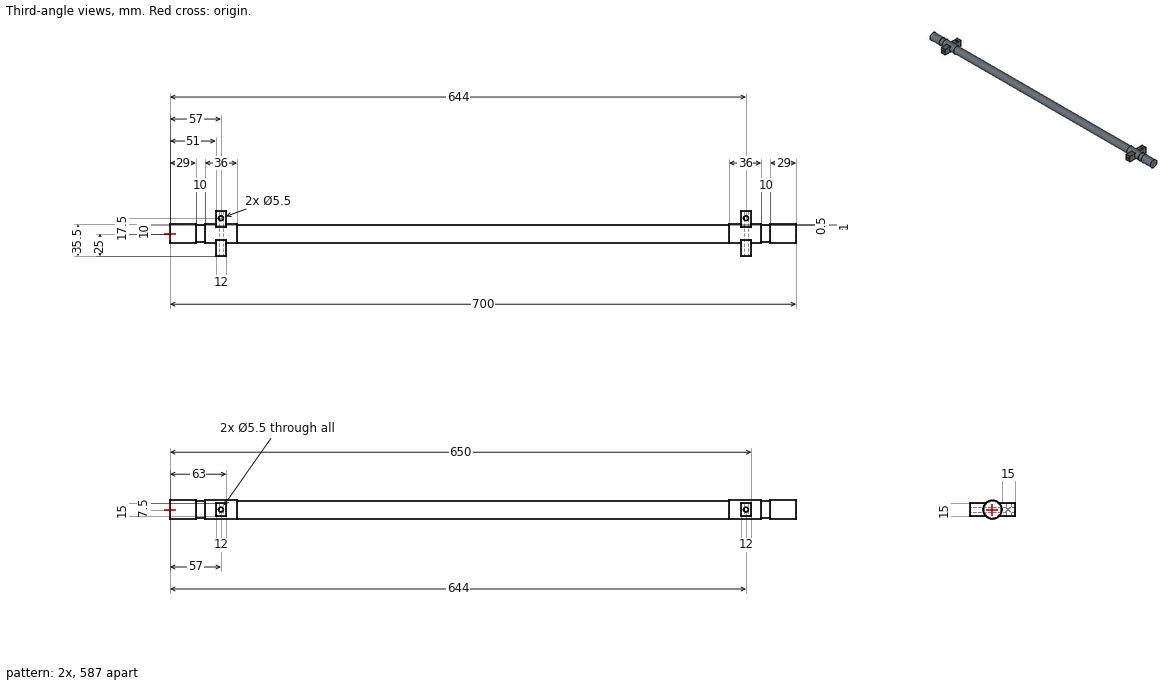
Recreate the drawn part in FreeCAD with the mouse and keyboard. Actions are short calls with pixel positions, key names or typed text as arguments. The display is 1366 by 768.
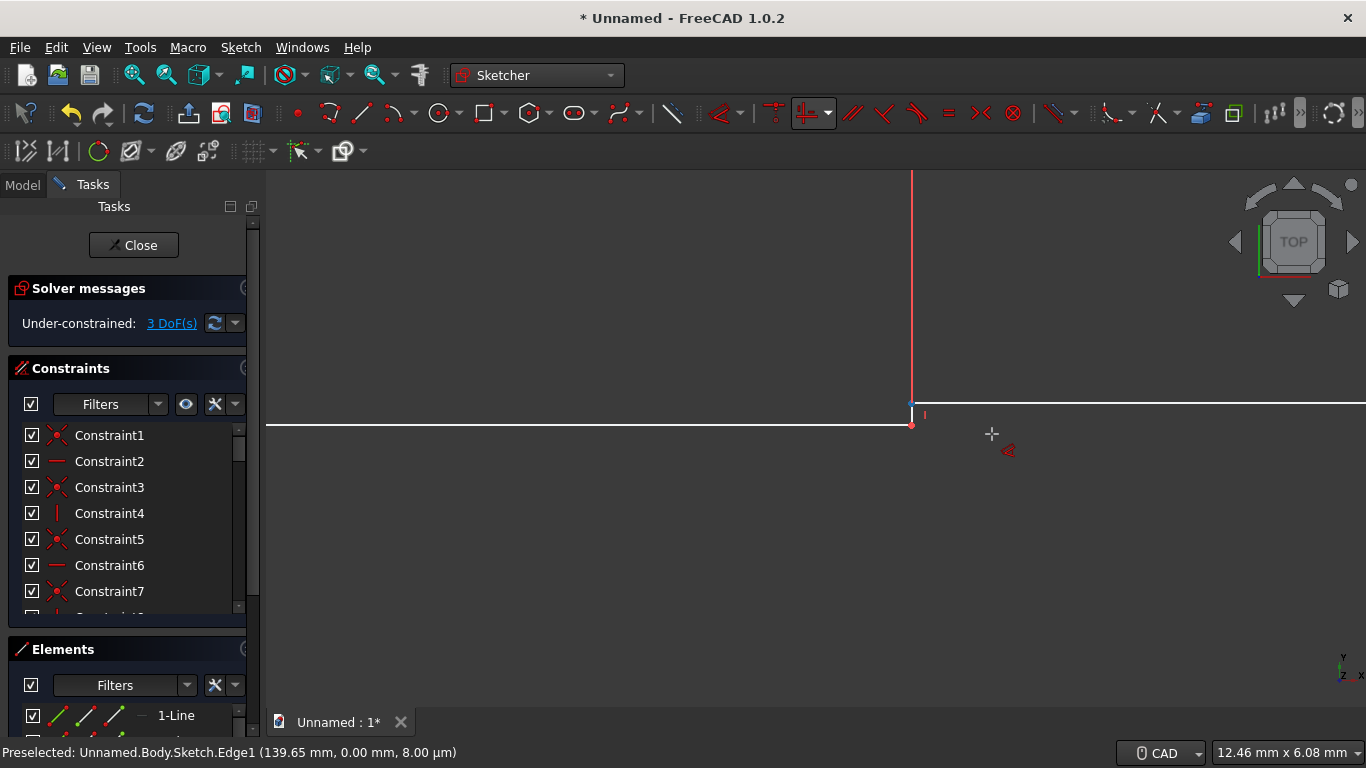
click(912, 414)
click(946, 419)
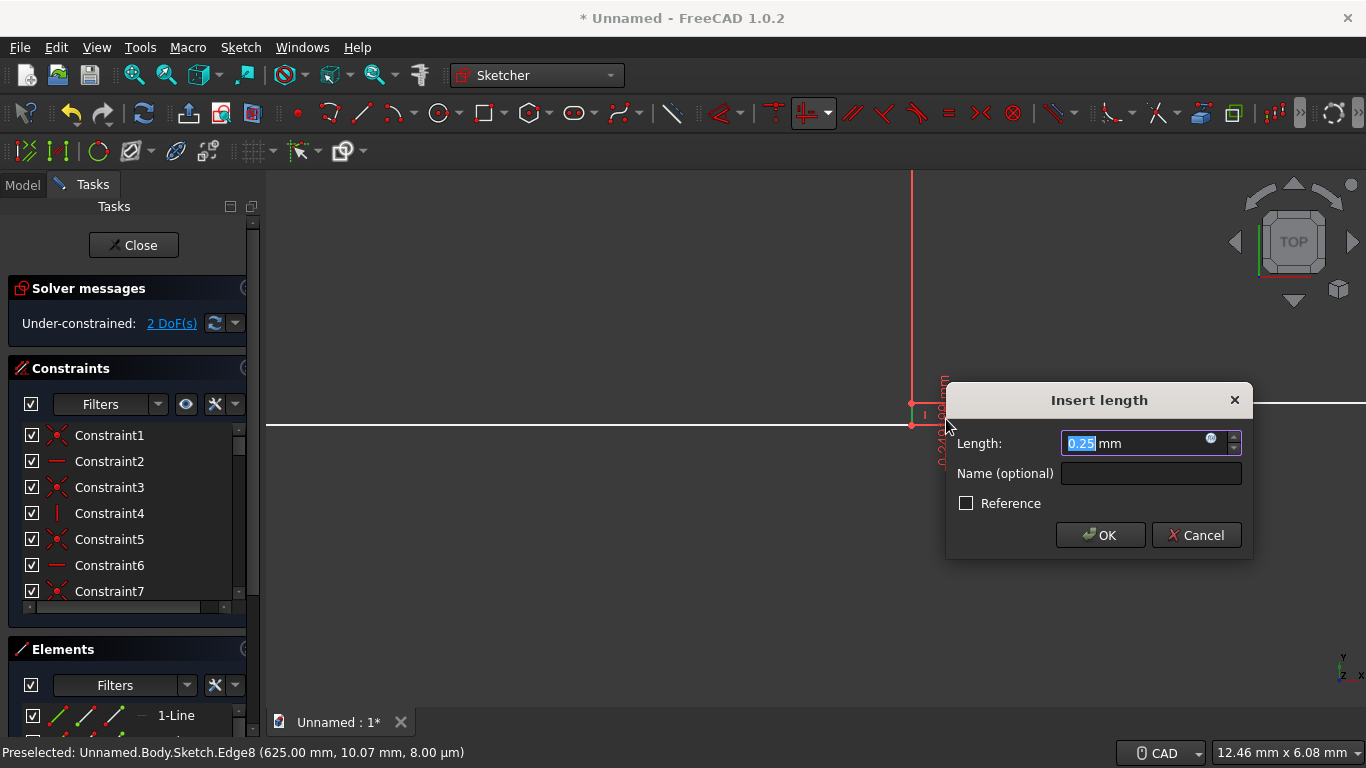
text(0.5)
key(Return)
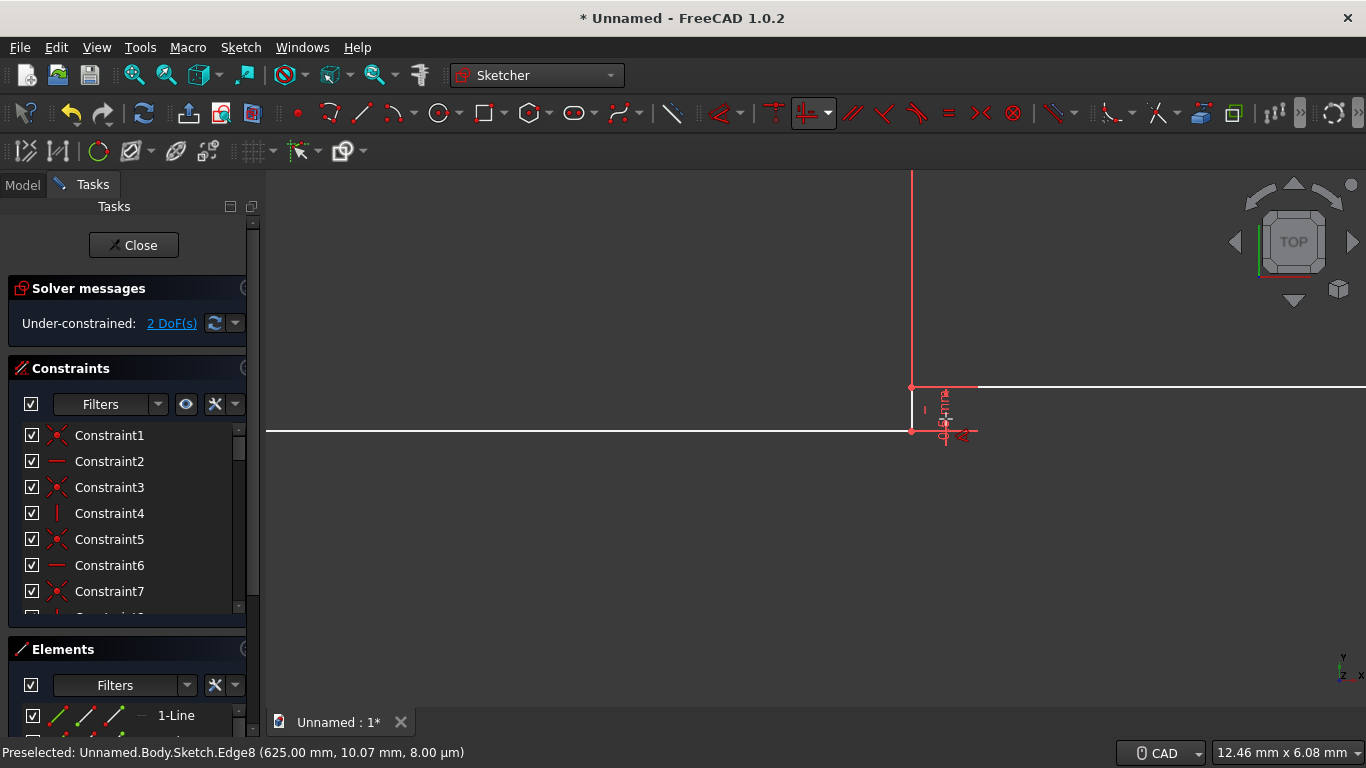
scroll(748, 438, down, 15)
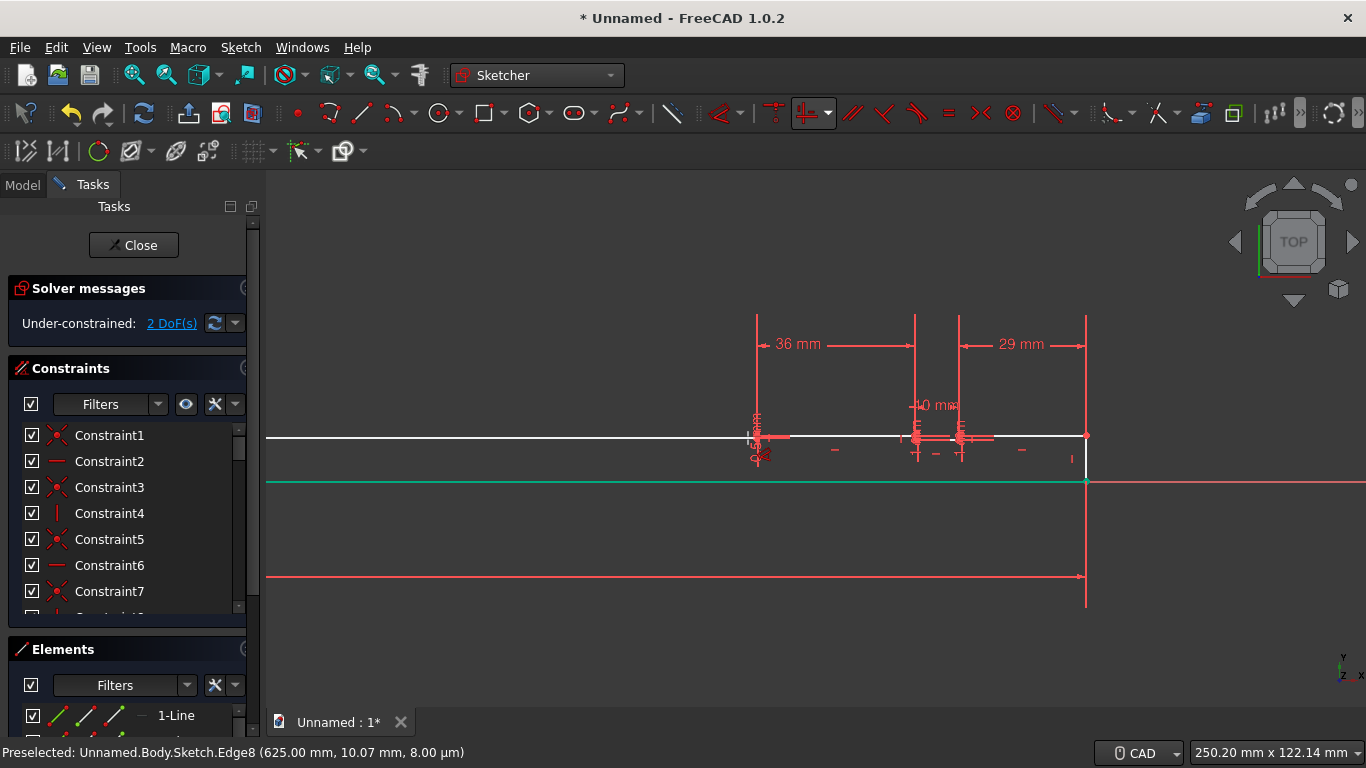
scroll(1051, 433, down, 8)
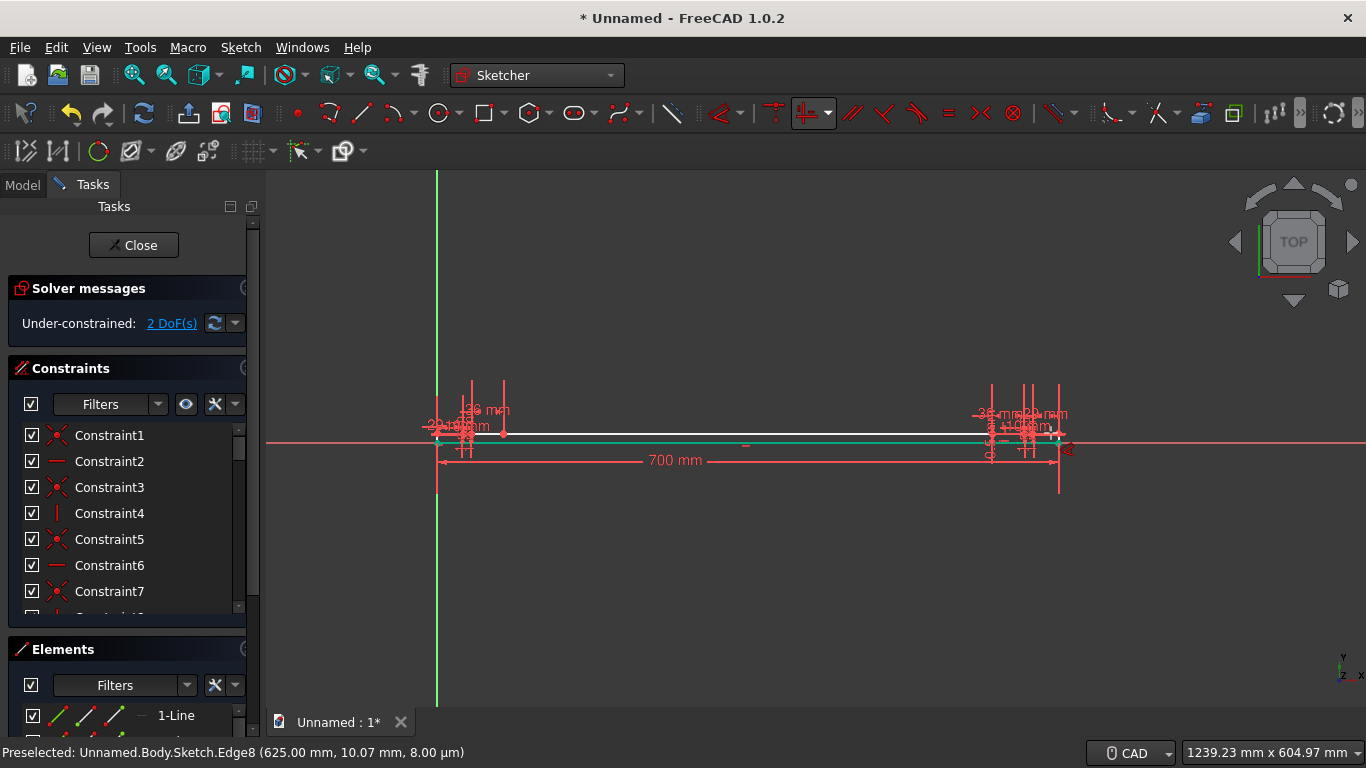
scroll(504, 434, up, 23)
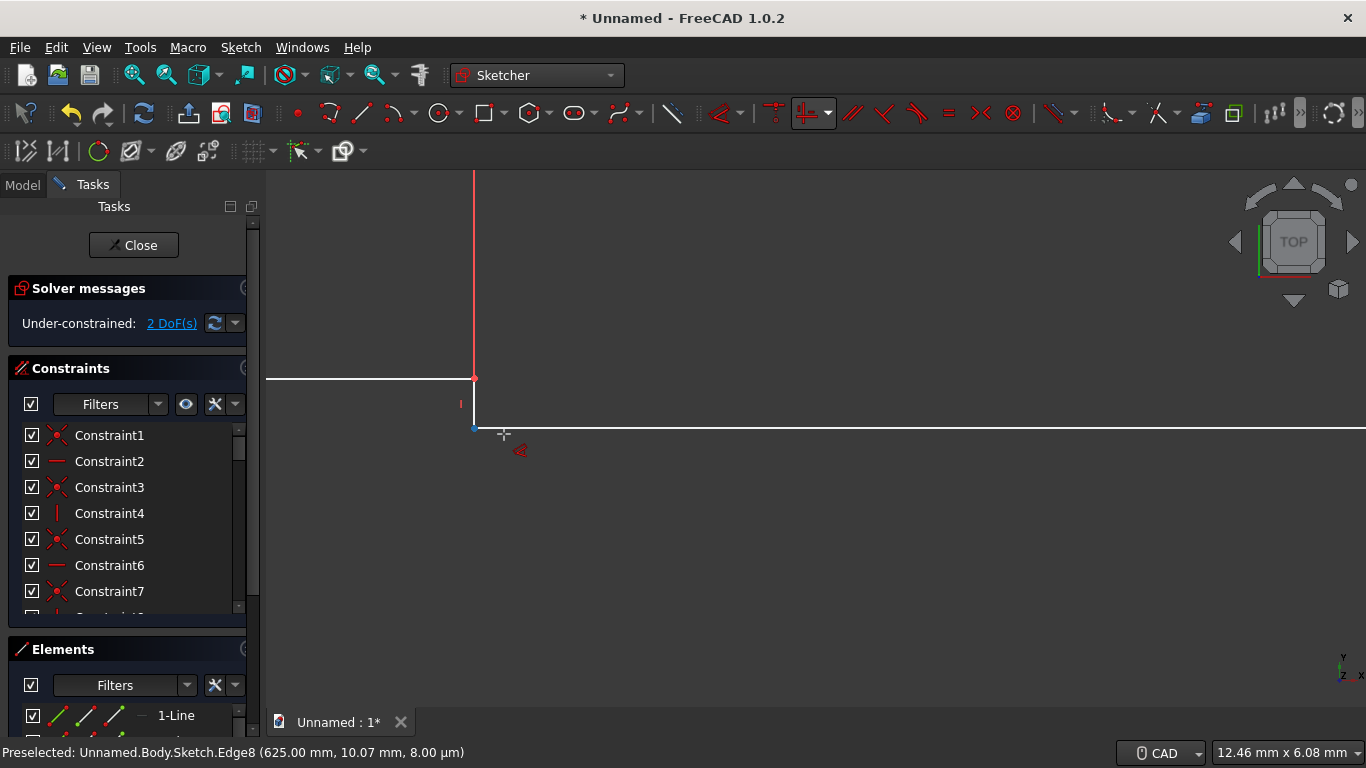
click(474, 413)
click(440, 403)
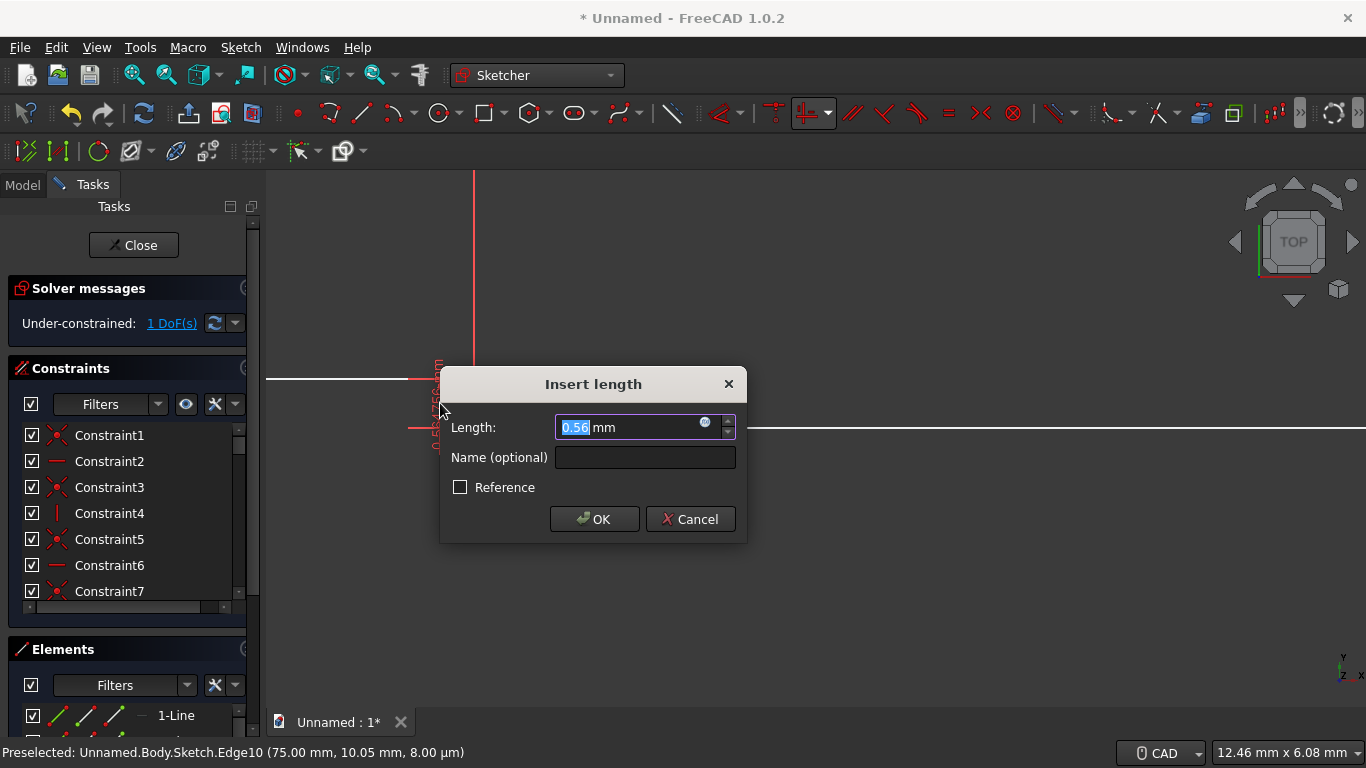
text(0.5)
key(Return)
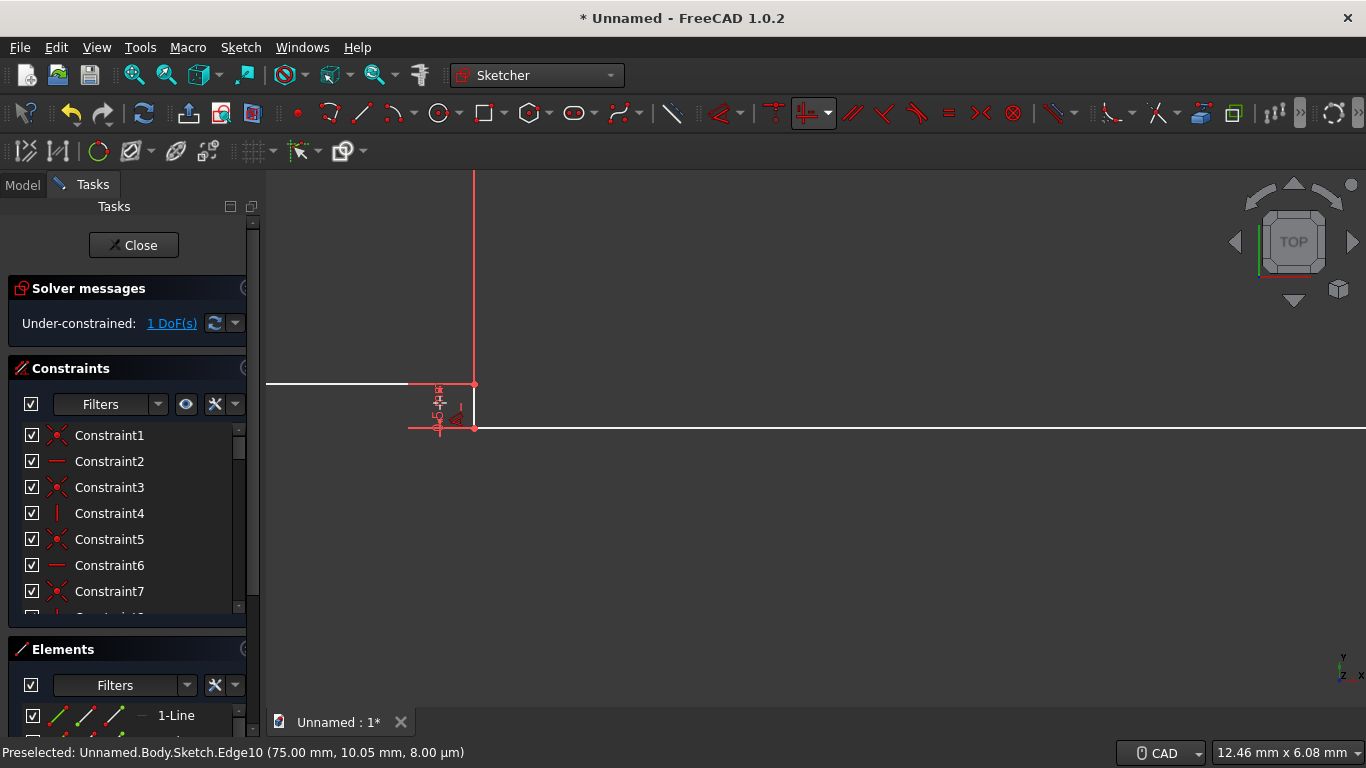
scroll(748, 438, down, 15)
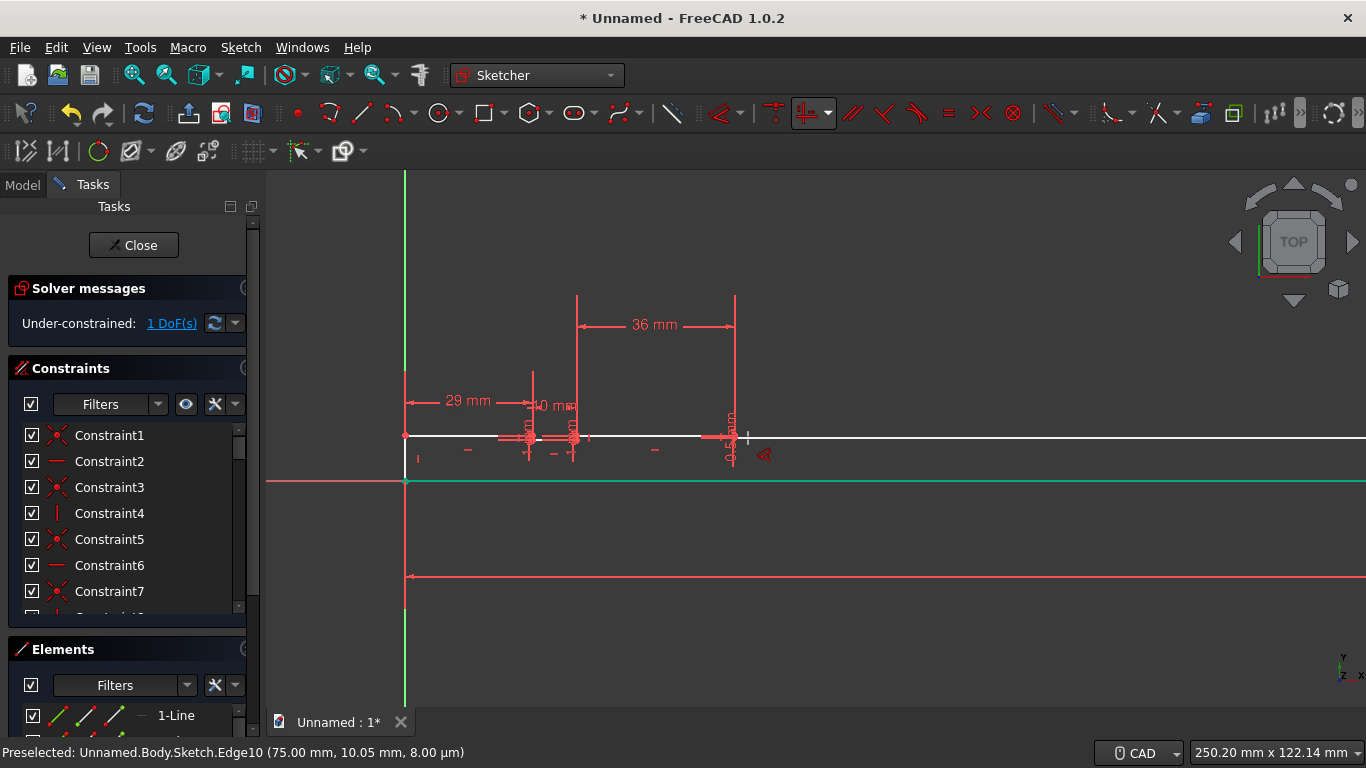
scroll(445, 433, down, 8)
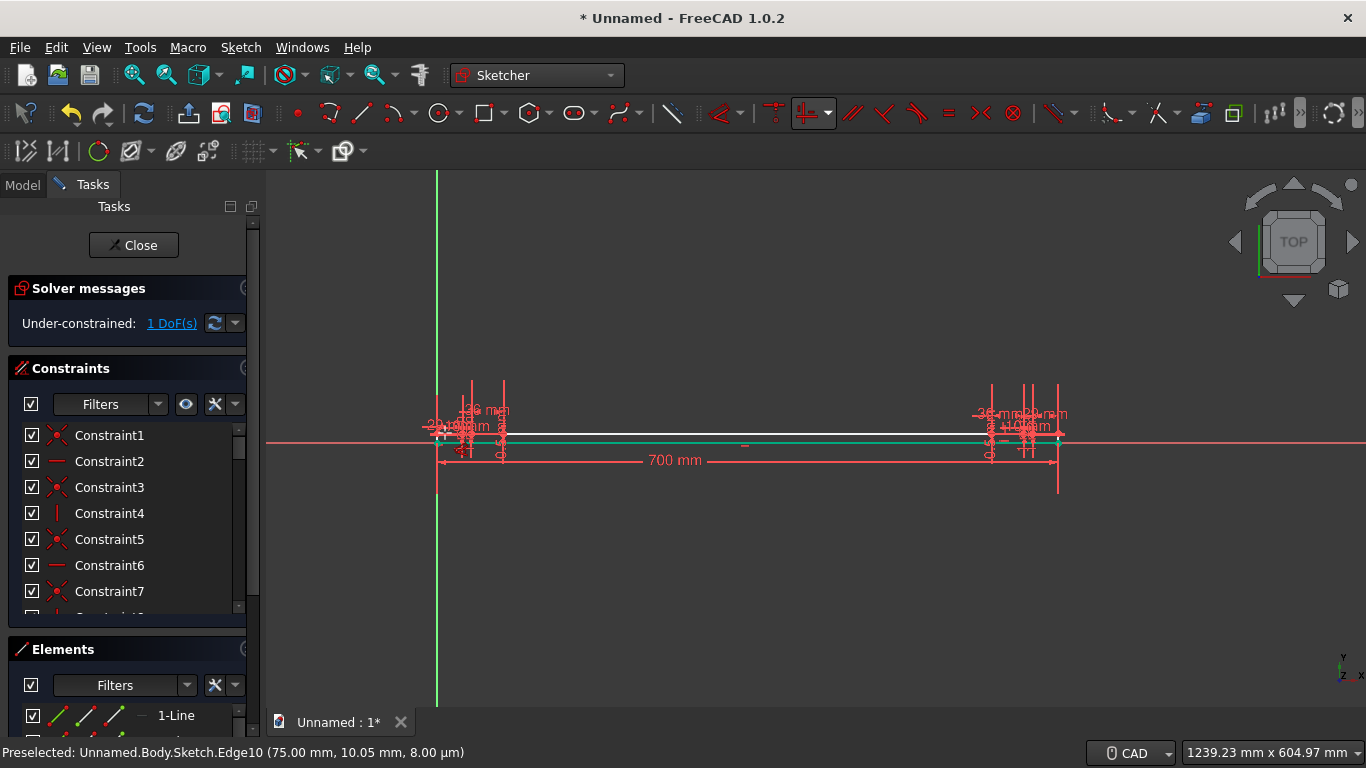
scroll(992, 434, up, 14)